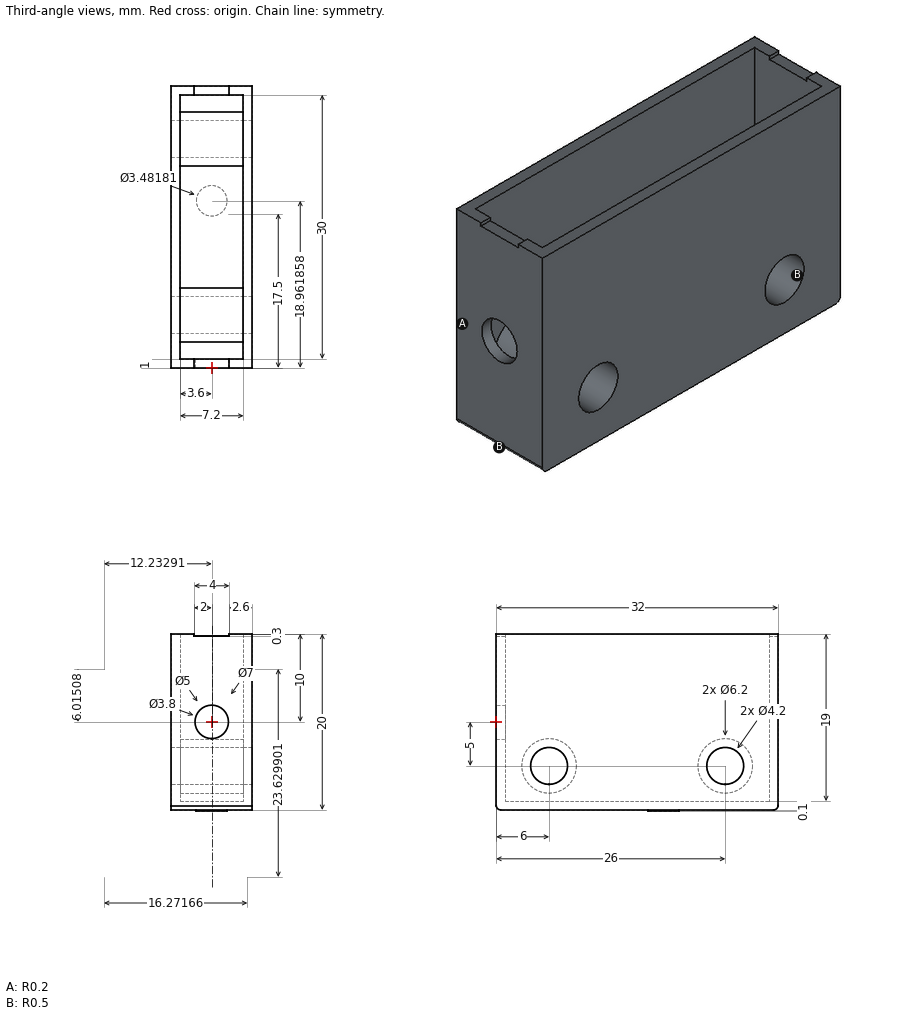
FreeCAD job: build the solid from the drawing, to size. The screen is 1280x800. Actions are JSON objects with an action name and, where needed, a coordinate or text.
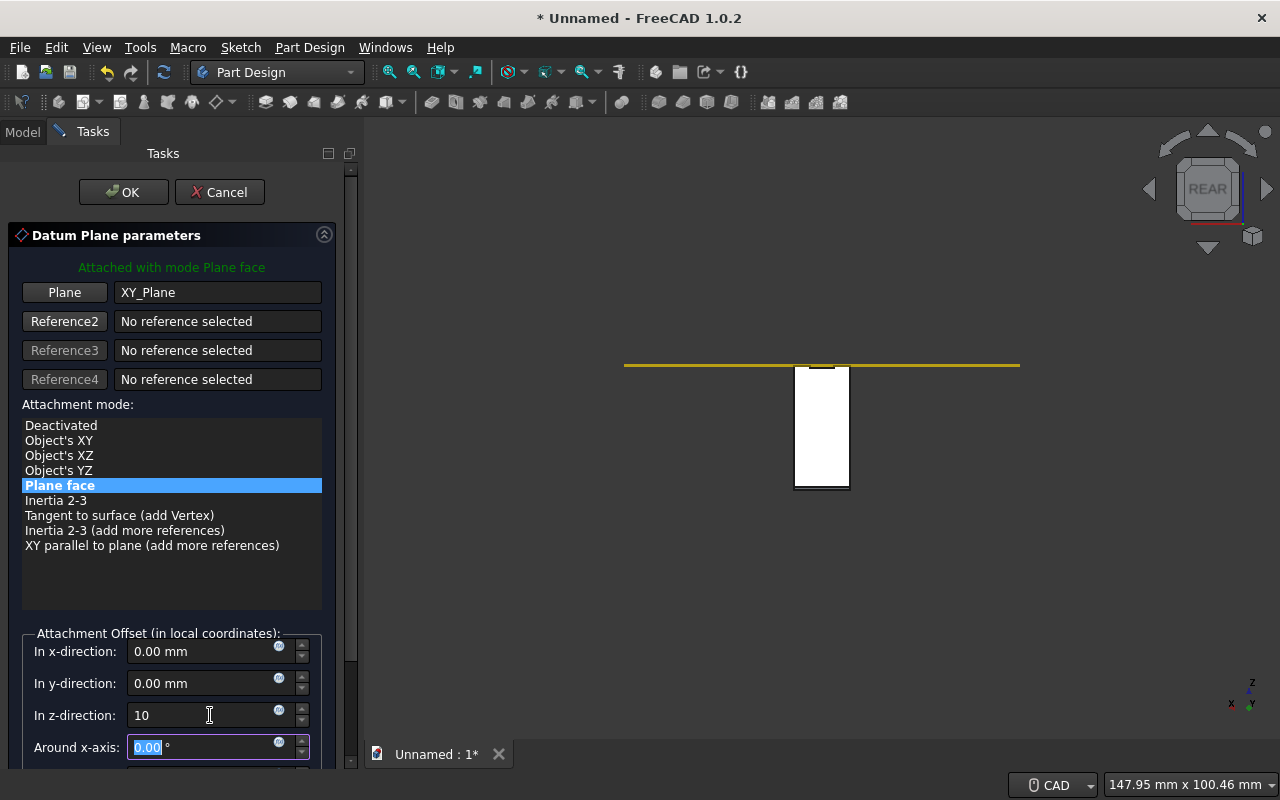
{"action": "left_click", "coordinate": [124, 192]}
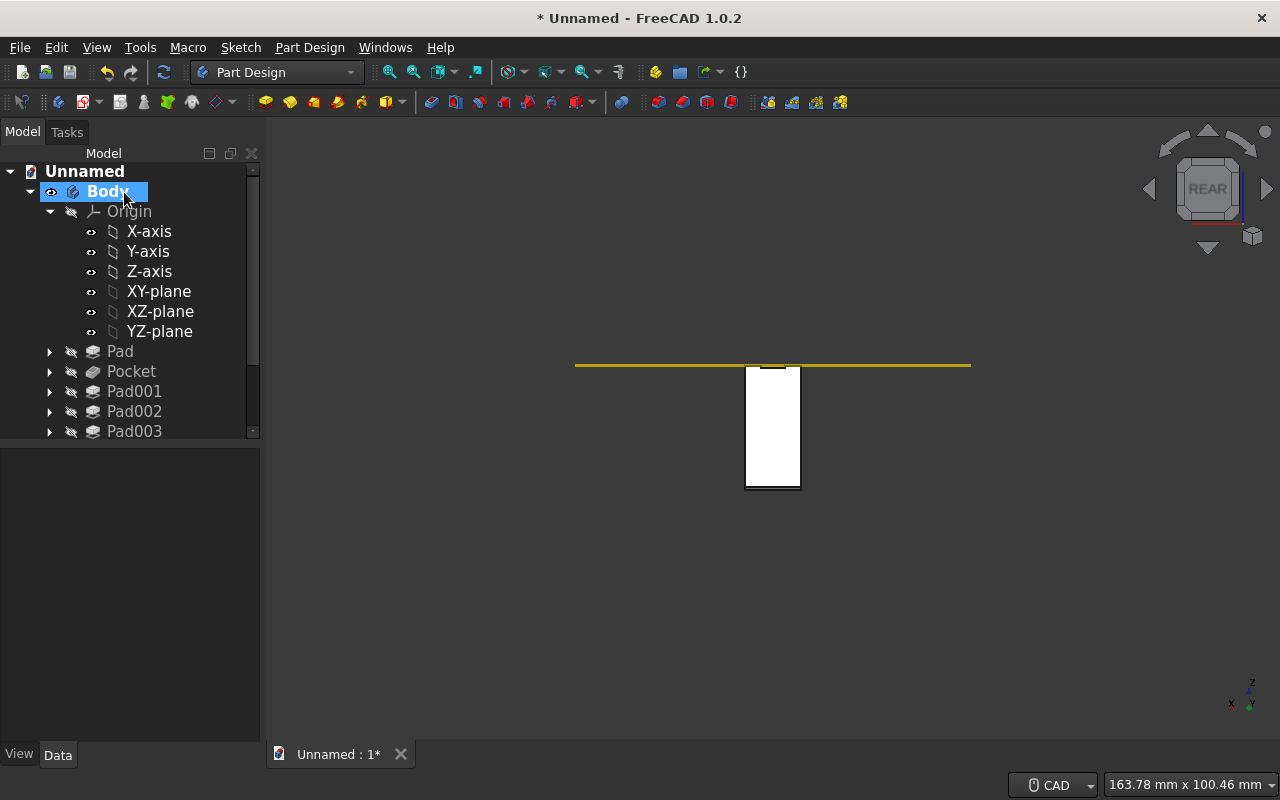
{"action": "scroll", "coordinate": [100, 307], "scroll_direction": "down", "scroll_amount": 3}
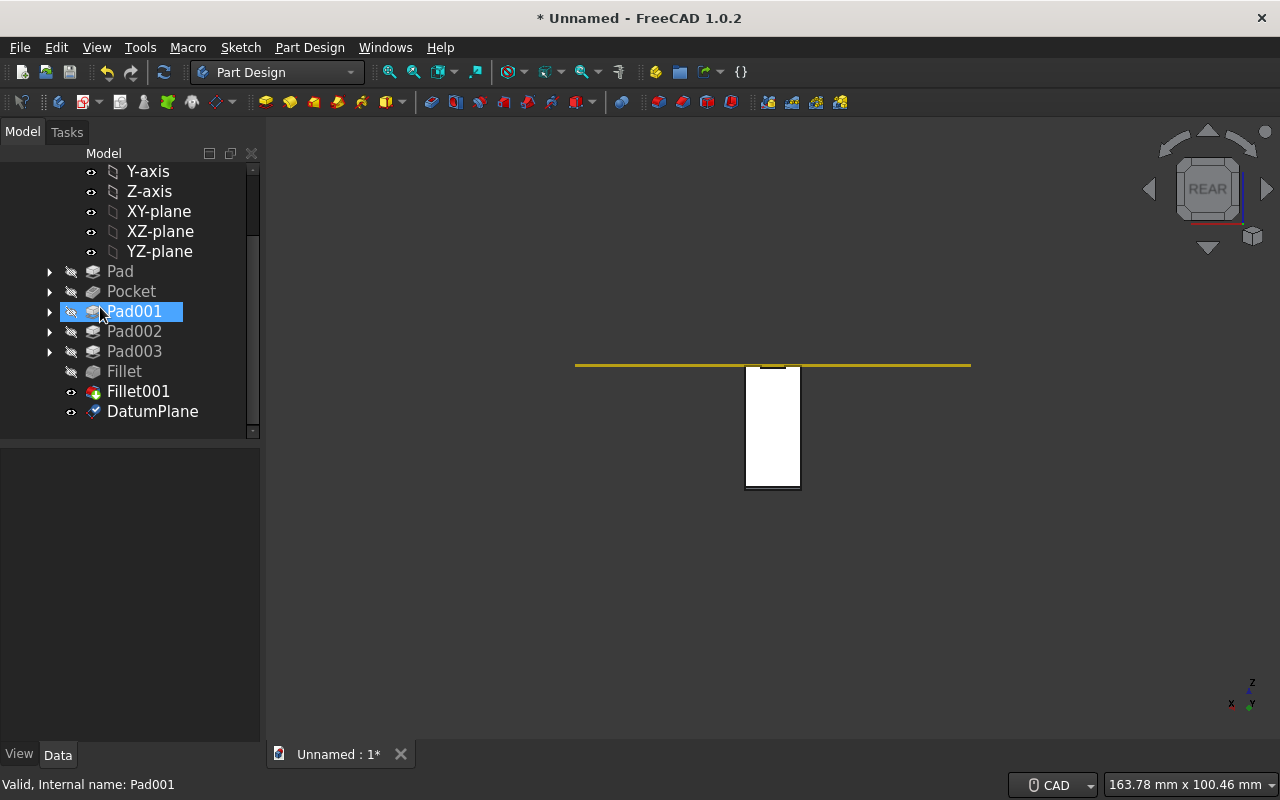
{"action": "left_click", "coordinate": [116, 412]}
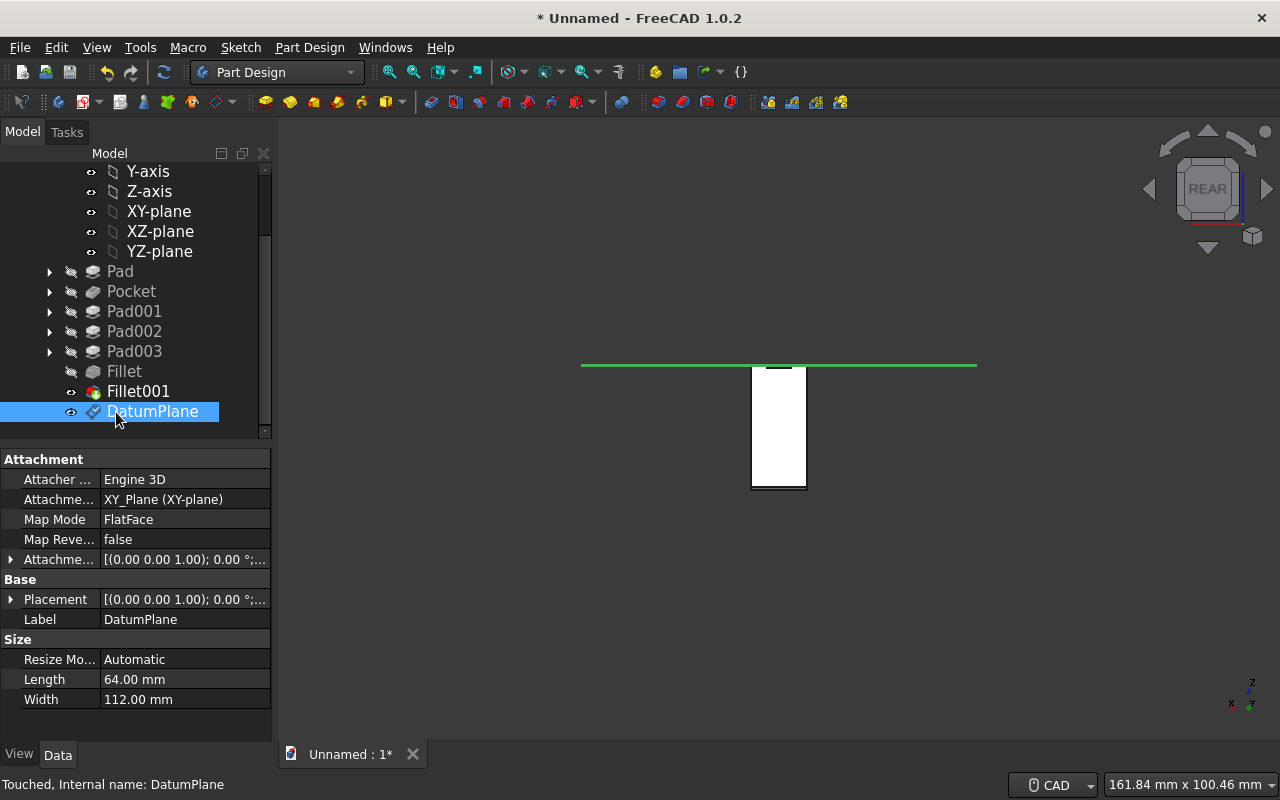
{"action": "left_click", "coordinate": [84, 102]}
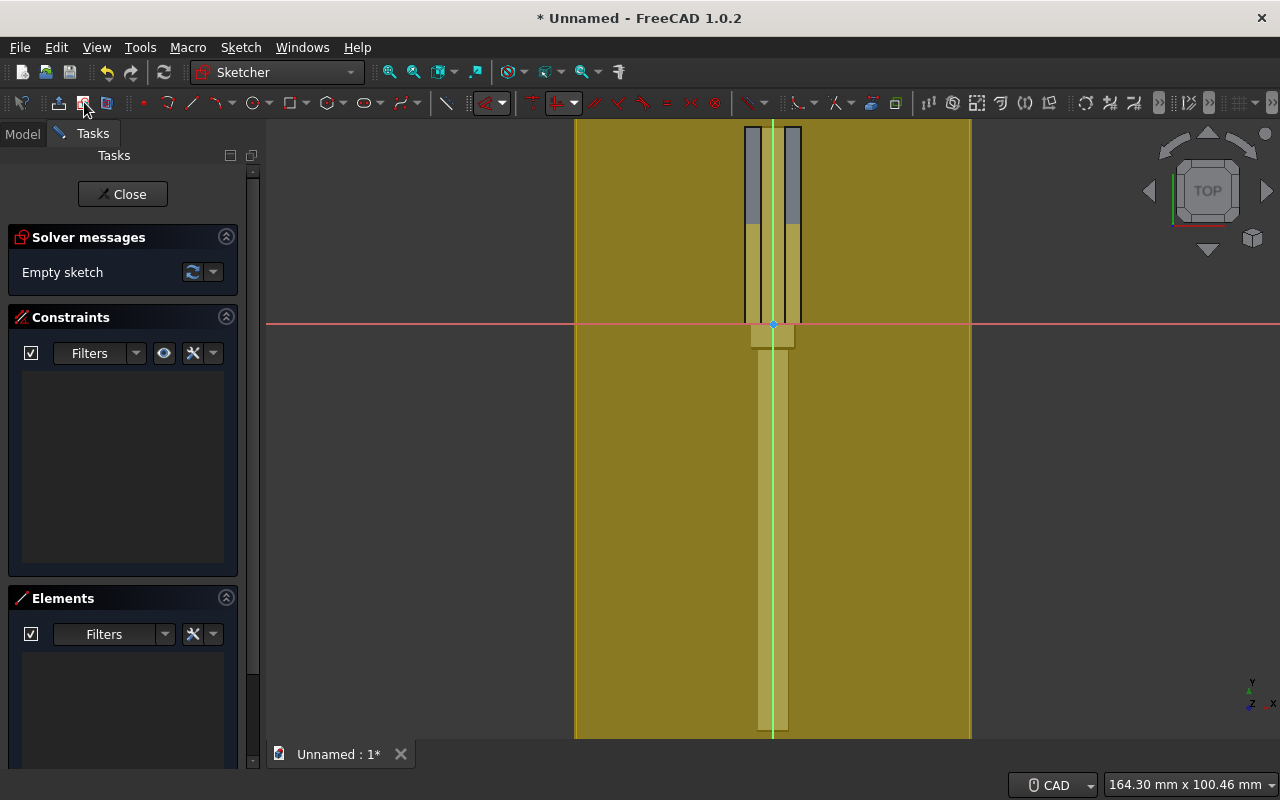
{"action": "scroll", "coordinate": [704, 429], "scroll_direction": "down", "scroll_amount": 5}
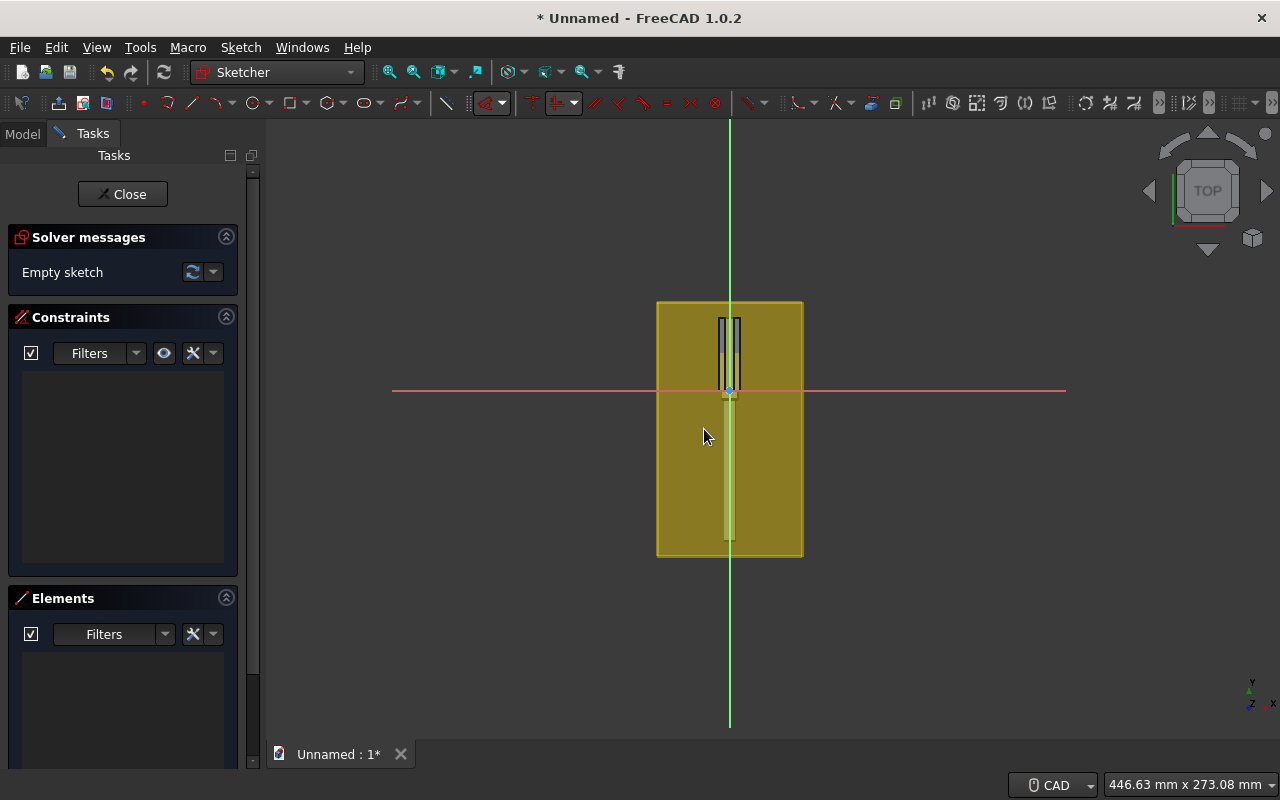
{"action": "scroll", "coordinate": [735, 341], "scroll_direction": "up", "scroll_amount": 9}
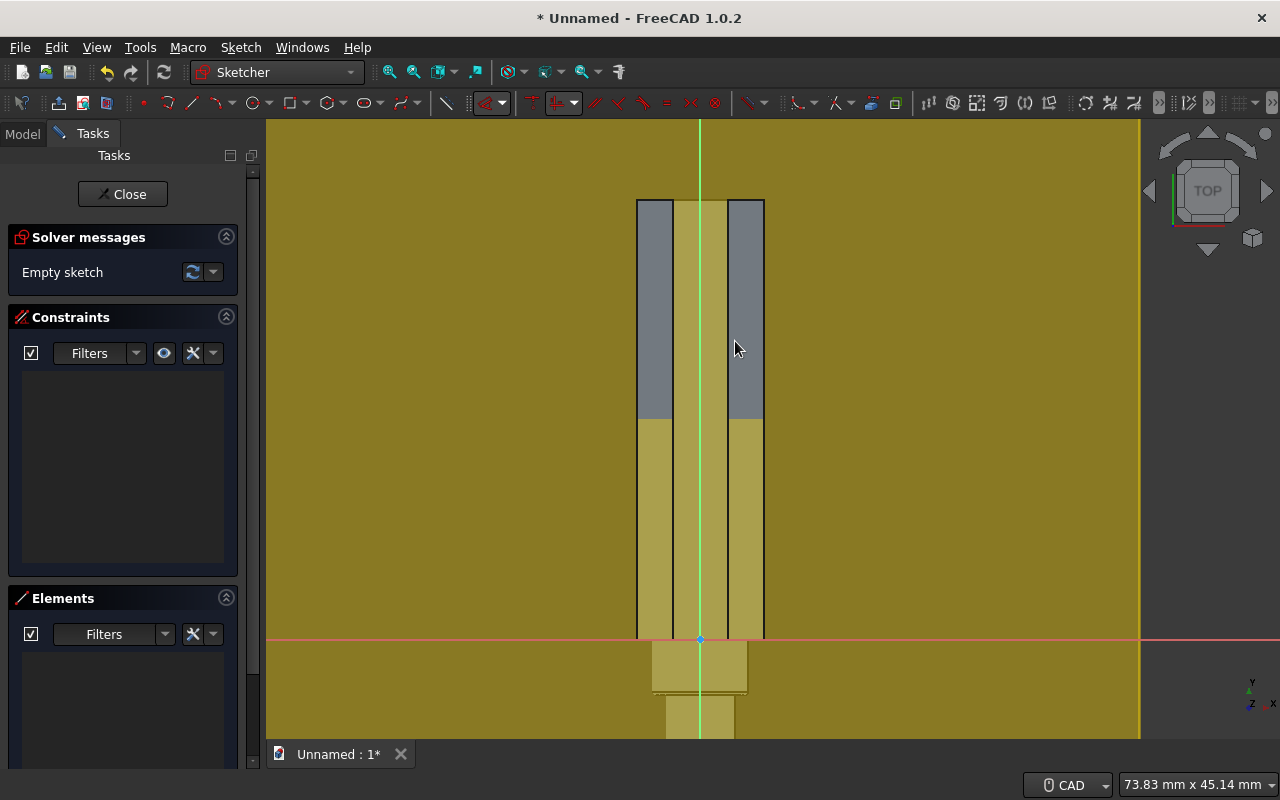
{"action": "left_click", "coordinate": [290, 104]}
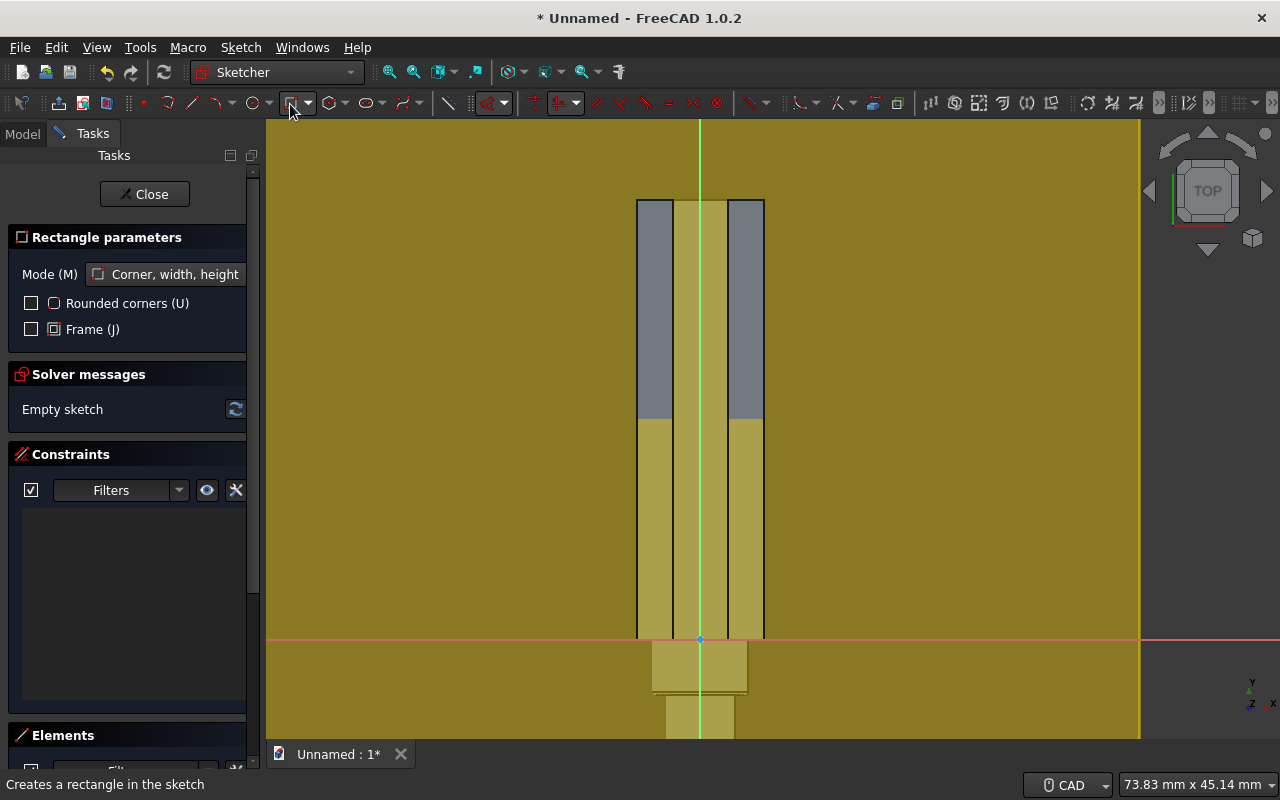
{"action": "left_click", "coordinate": [651, 214]}
{"action": "mouse_move", "coordinate": [750, 626]}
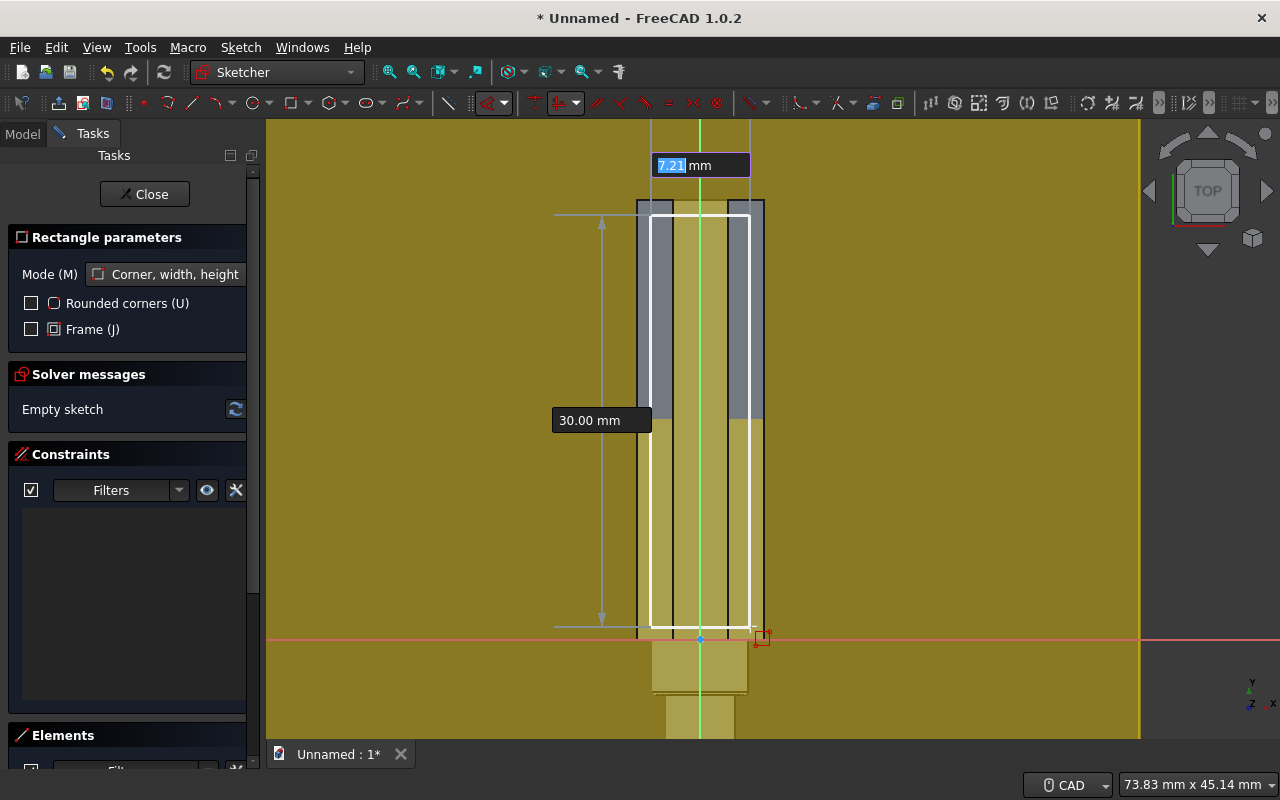
{"action": "type", "text": "7.2"}
{"action": "key", "text": "Tab"}
{"action": "type", "text": "30"}
{"action": "key", "text": "Return"}
{"action": "key", "text": "Escape"}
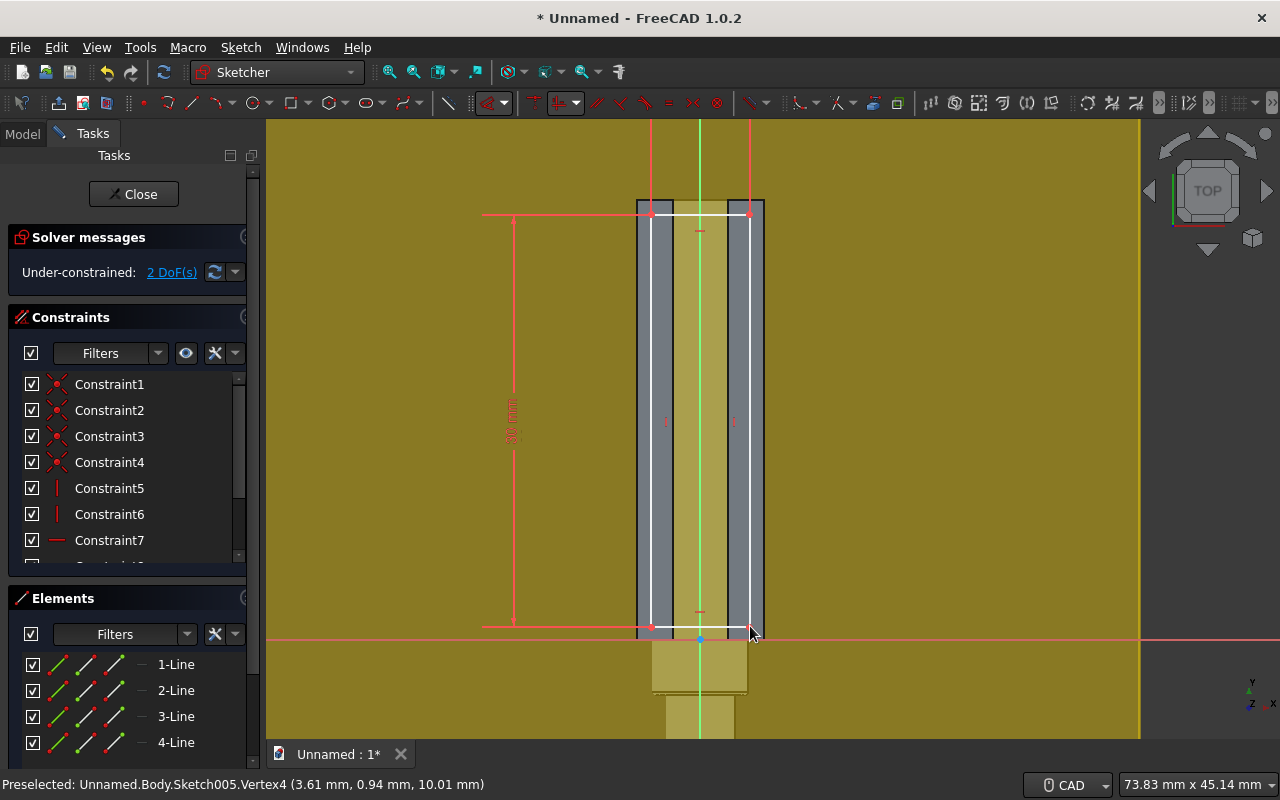
{"action": "scroll", "coordinate": [651, 627], "scroll_direction": "up", "scroll_amount": 6}